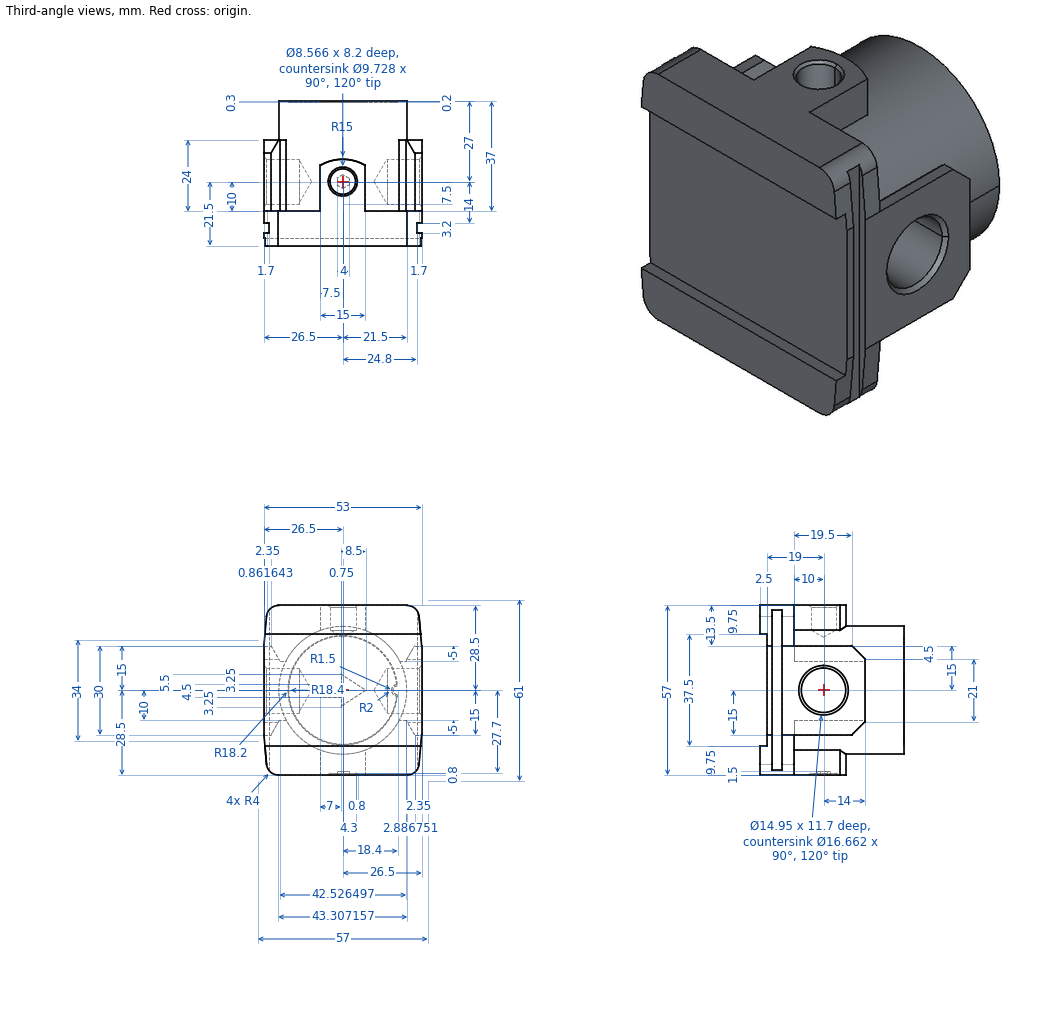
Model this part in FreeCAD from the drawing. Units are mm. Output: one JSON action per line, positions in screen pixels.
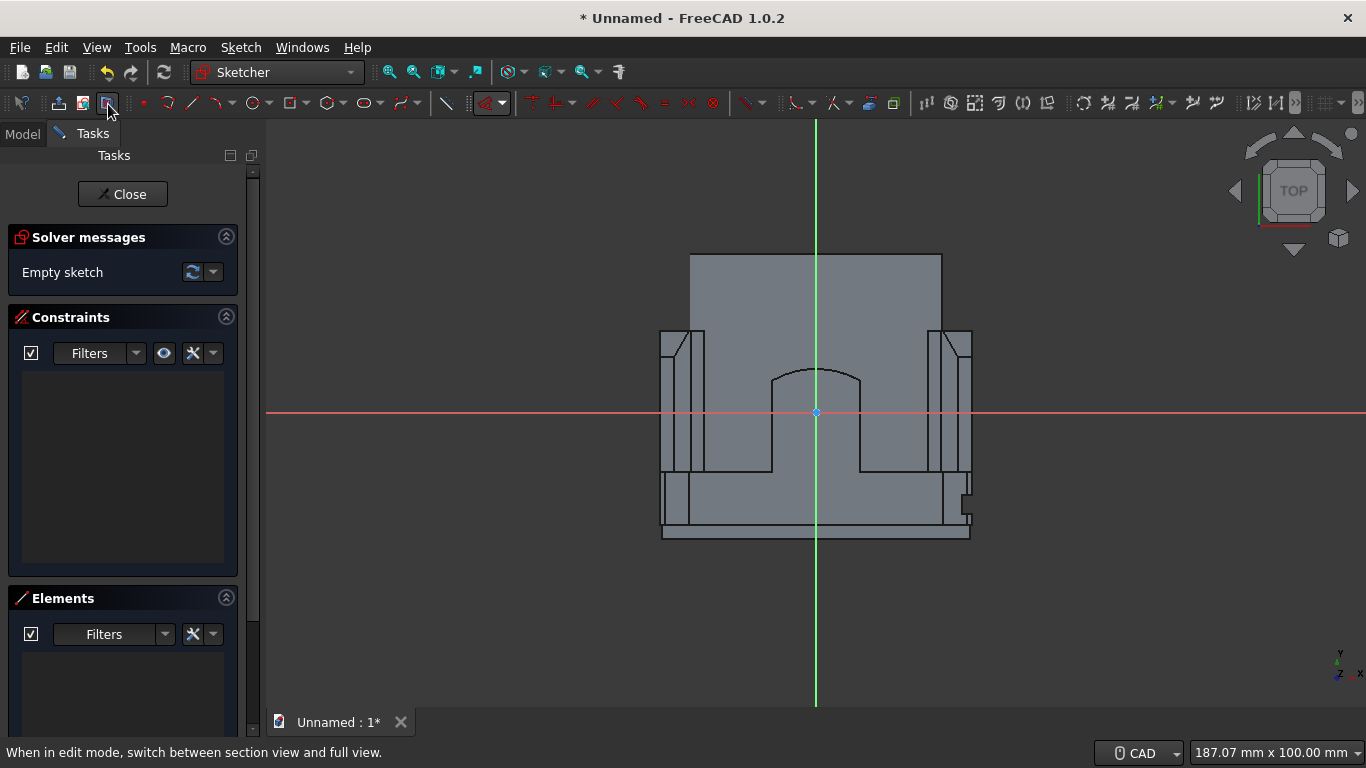
{"action": "scroll", "coordinate": [661, 510], "scroll_direction": "up", "scroll_amount": 15}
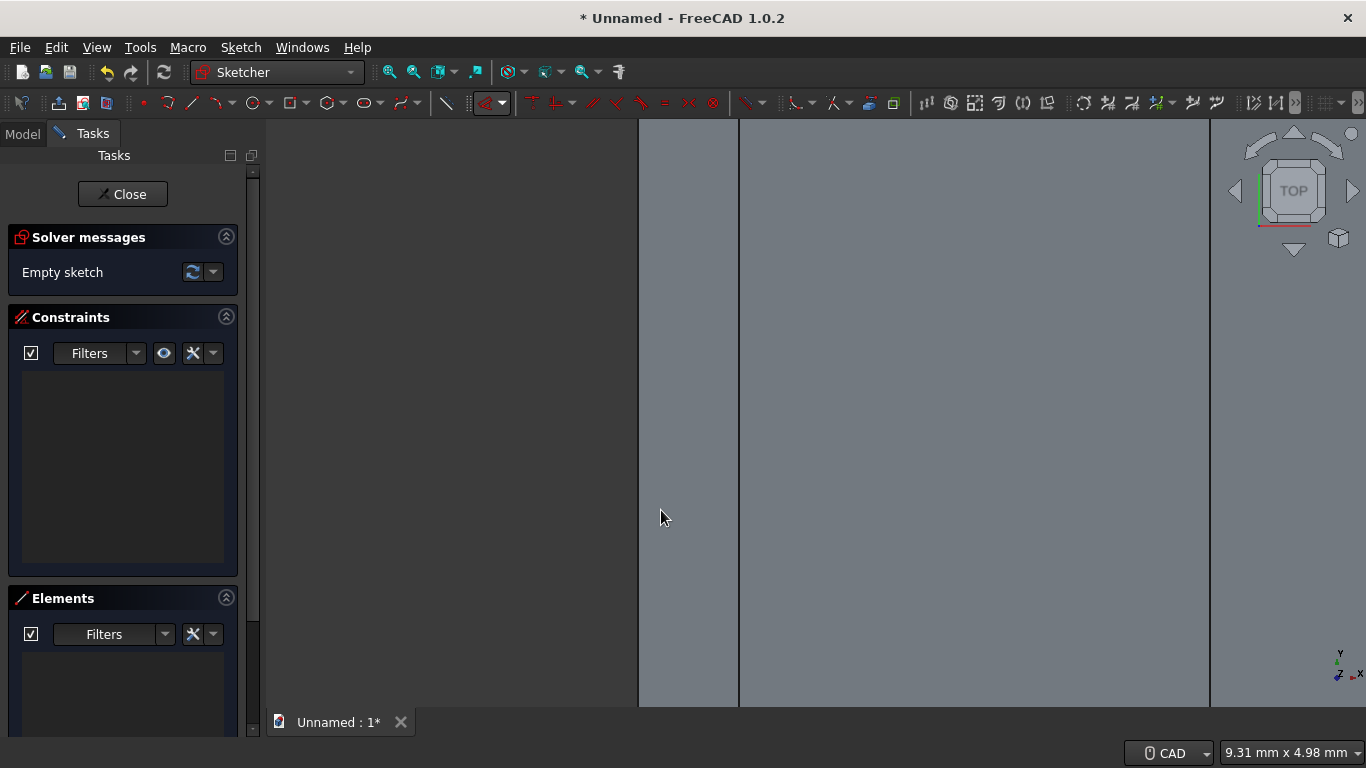
{"action": "key", "text": "g r"}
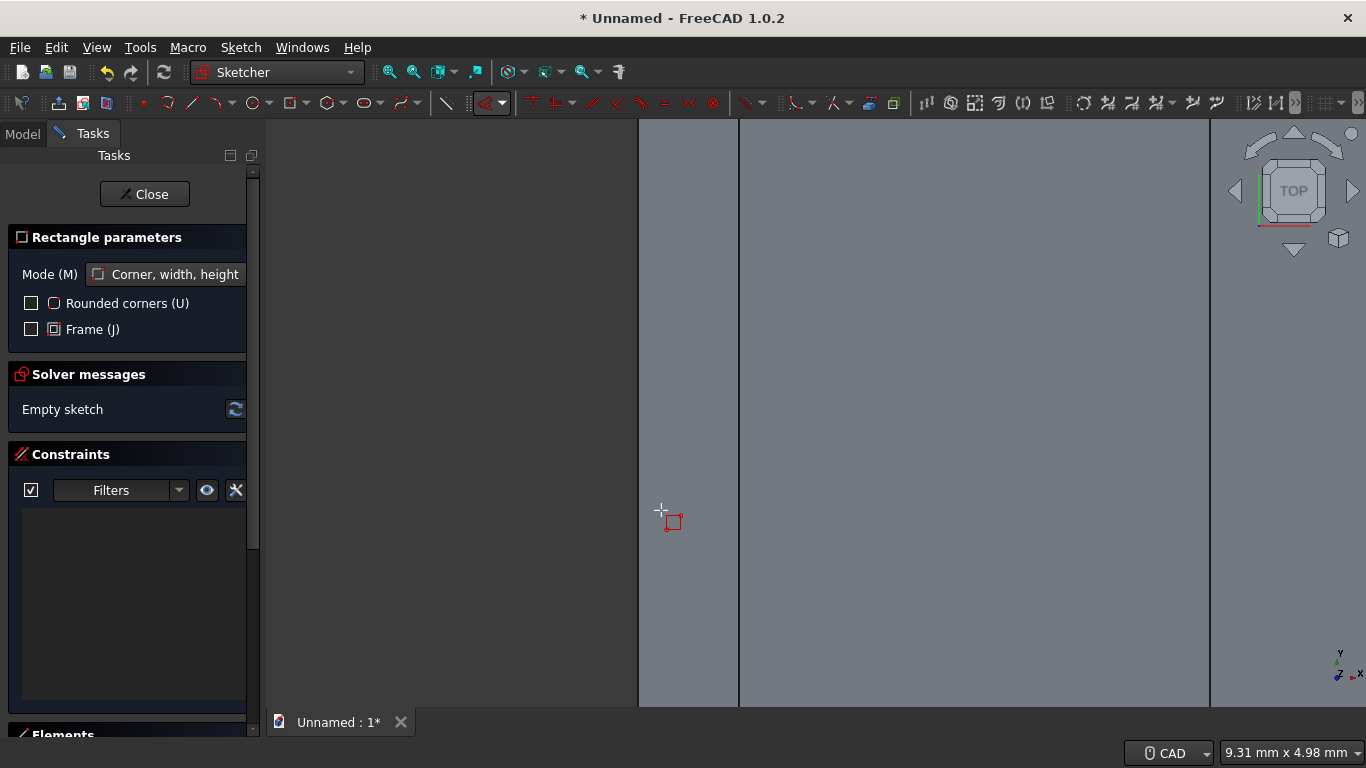
{"action": "left_click", "coordinate": [638, 202]}
{"action": "mouse_move", "coordinate": [838, 580]}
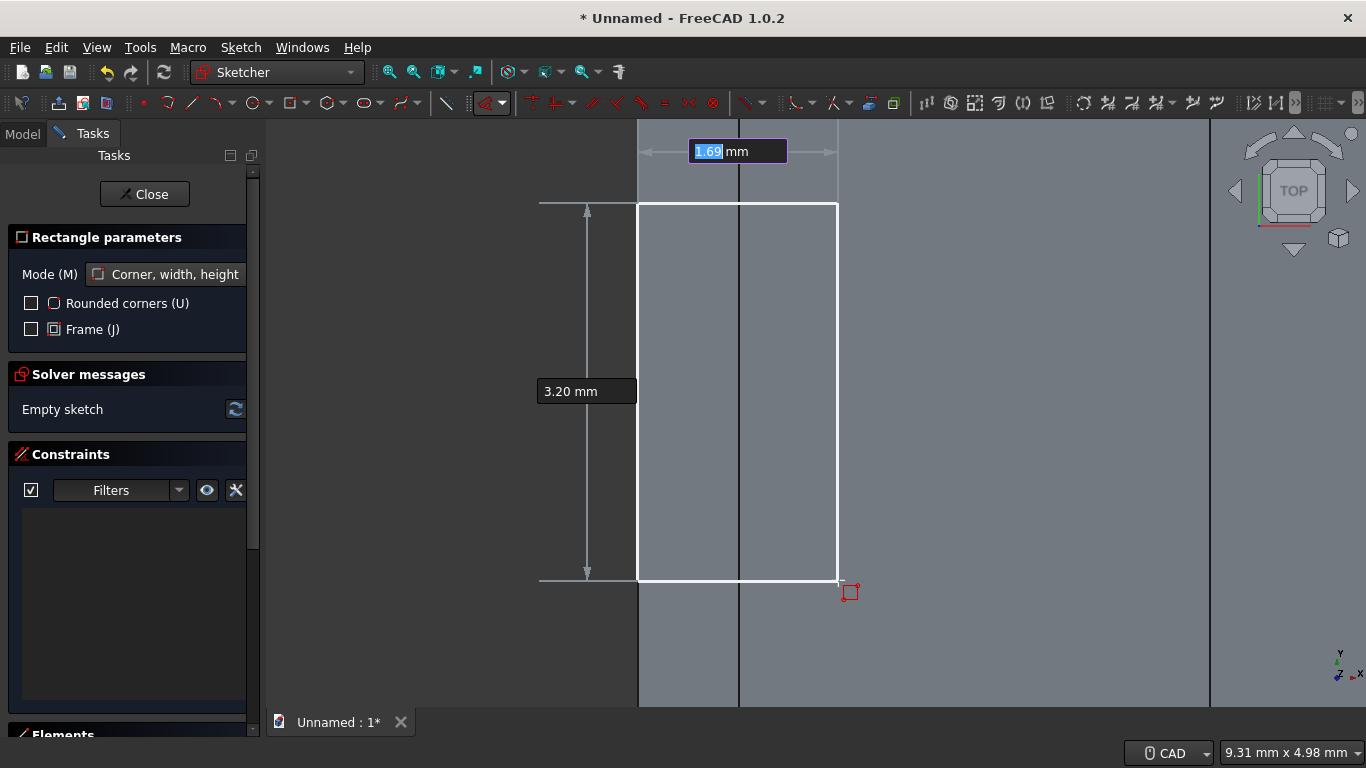
{"action": "type", "text": "1.7"}
{"action": "key", "text": "Tab"}
{"action": "type", "text": "3.2"}
{"action": "key", "text": "Return"}
{"action": "key", "text": "Escape"}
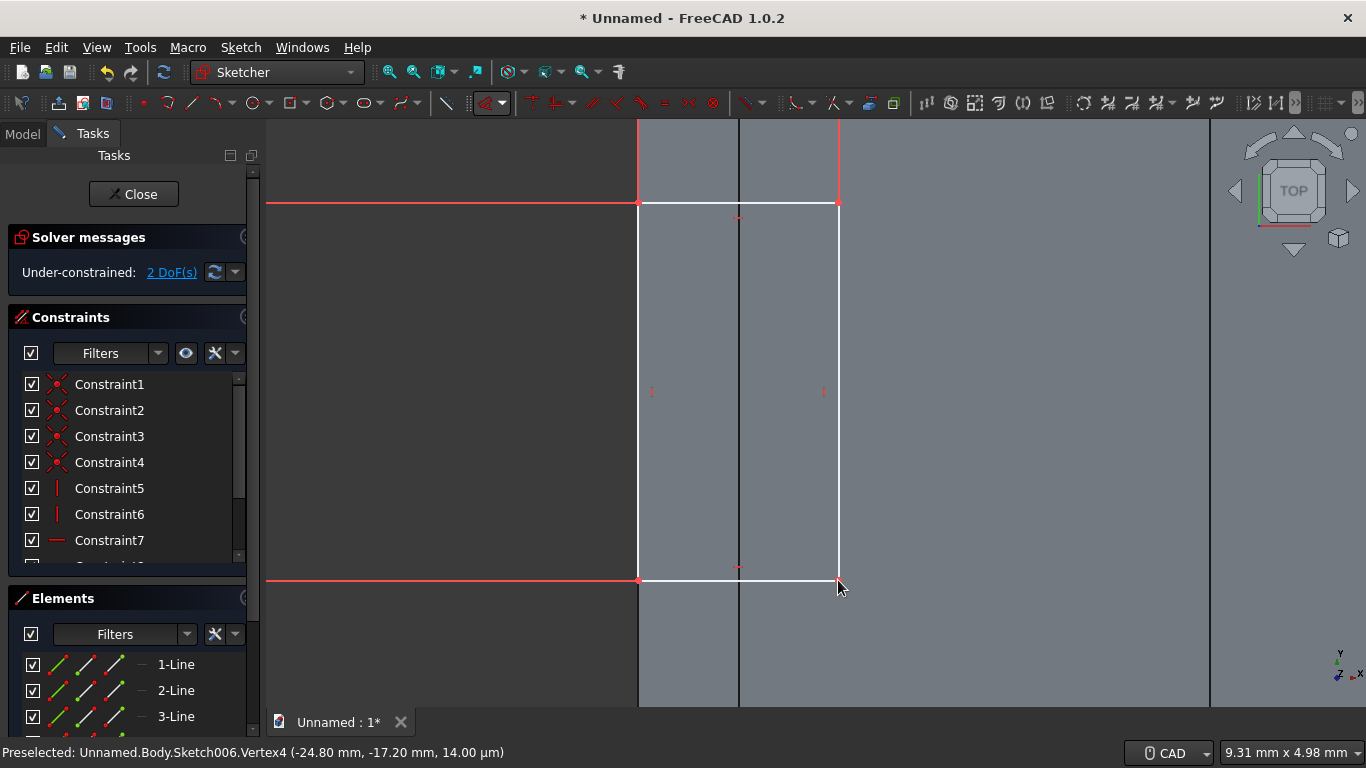
{"action": "left_click", "coordinate": [638, 203]}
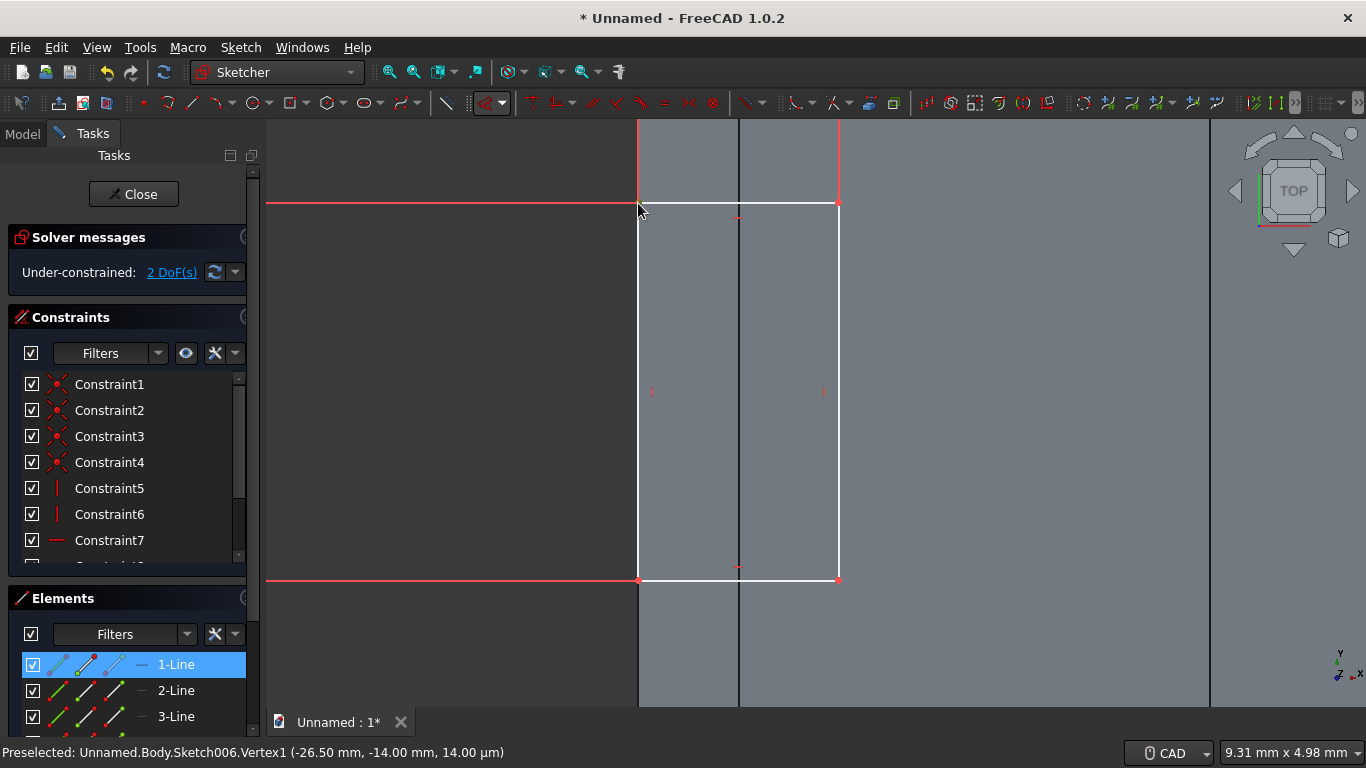
{"action": "left_click", "coordinate": [504, 104]}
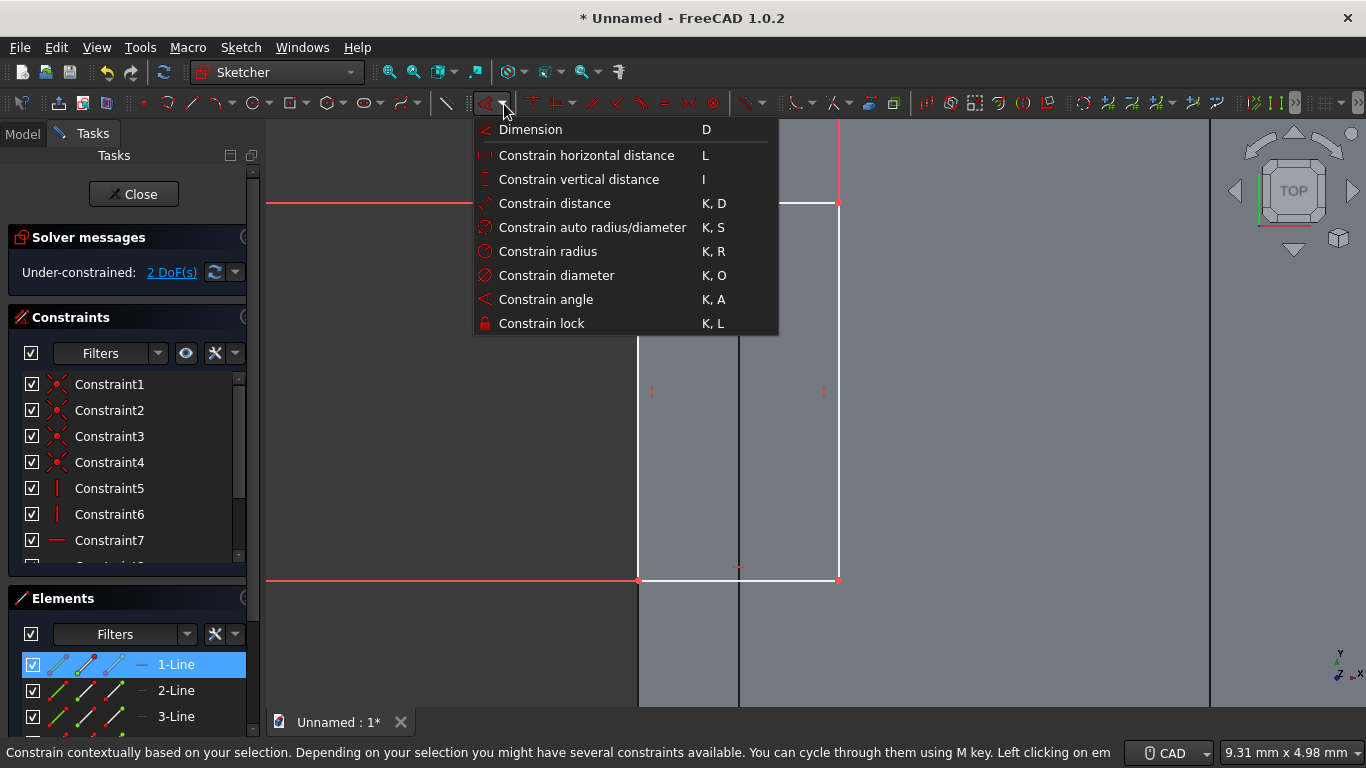
{"action": "left_click", "coordinate": [626, 179]}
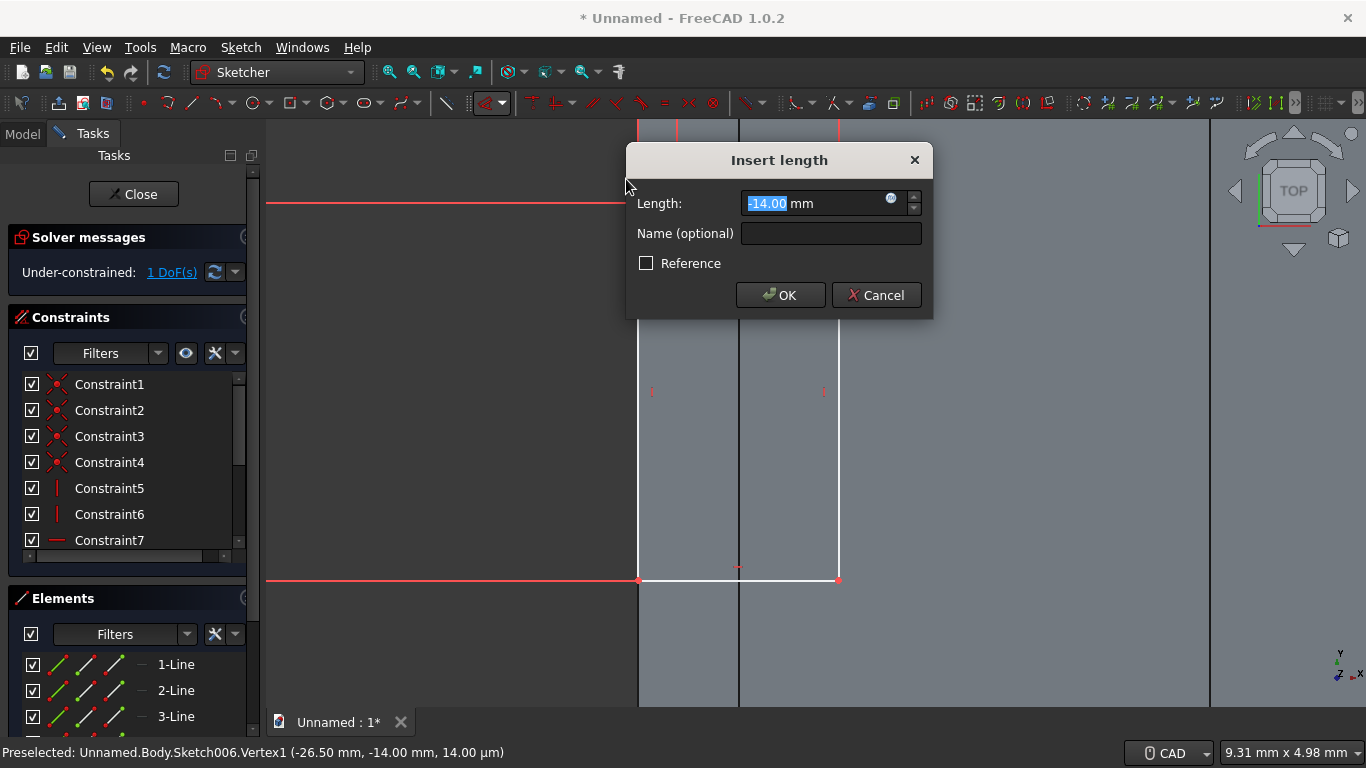
{"action": "type", "text": "-14"}
{"action": "key", "text": "Return"}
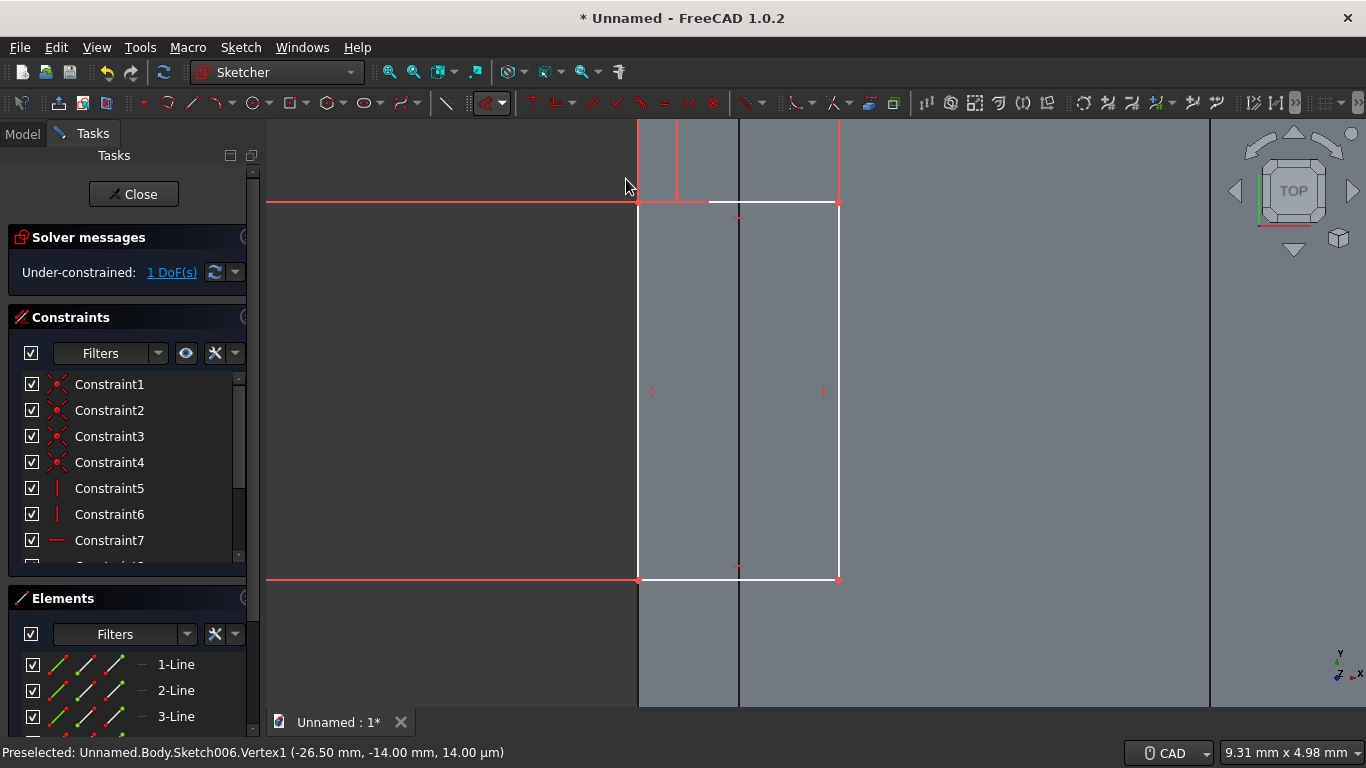
{"action": "left_click", "coordinate": [638, 202]}